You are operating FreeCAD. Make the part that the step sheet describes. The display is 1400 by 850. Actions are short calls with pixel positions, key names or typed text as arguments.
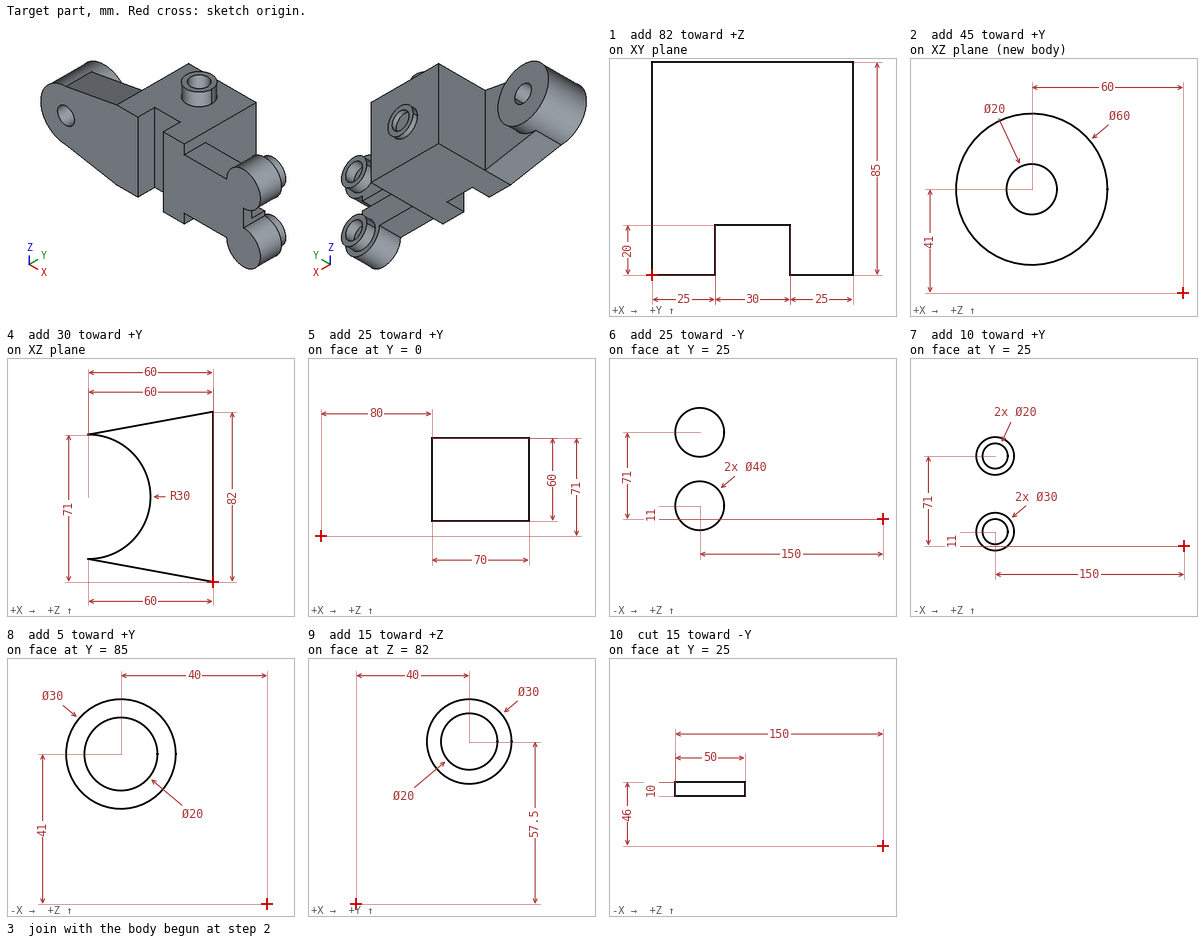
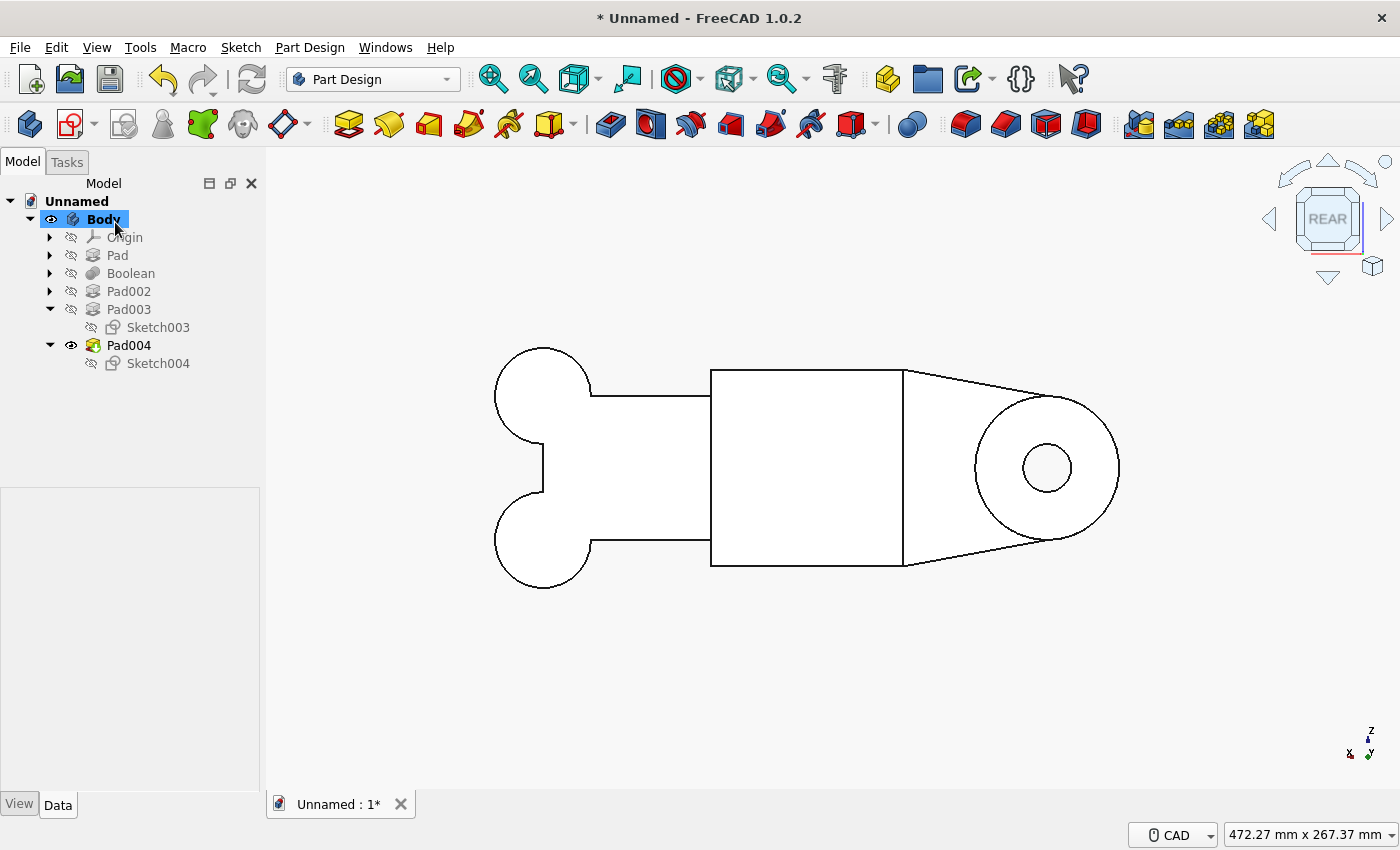
click(634, 467)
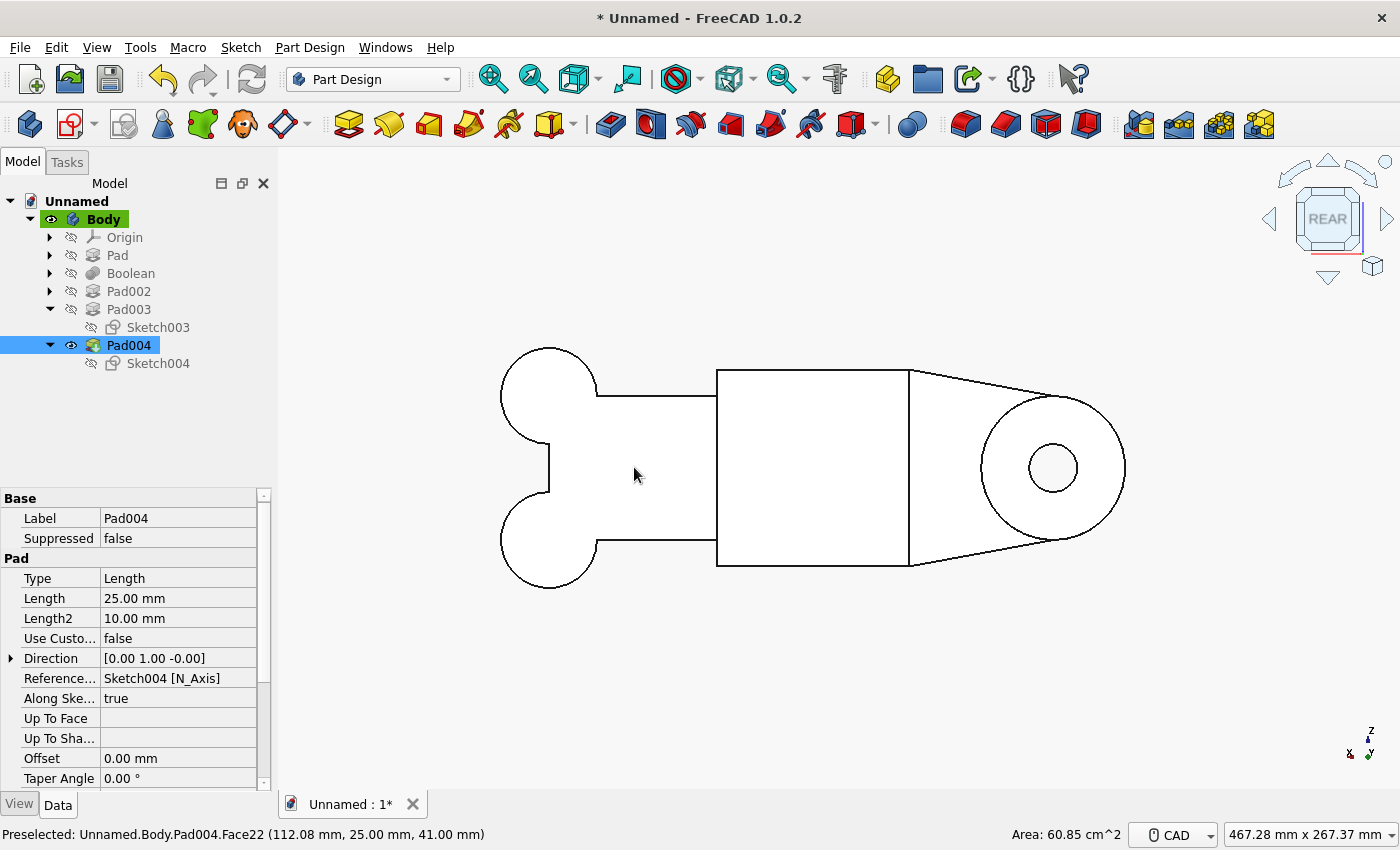
click(70, 124)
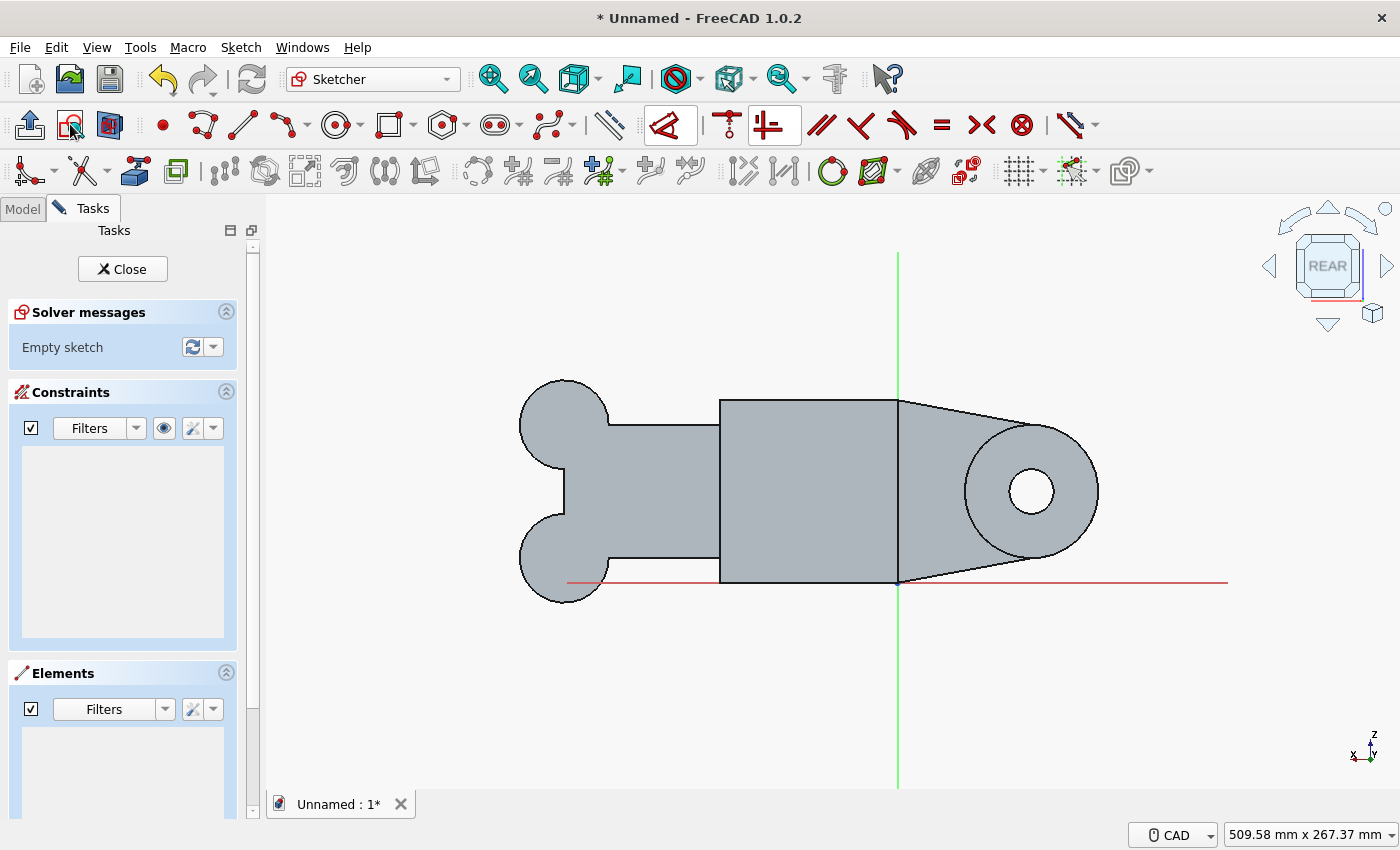
scroll(653, 492, up, 3)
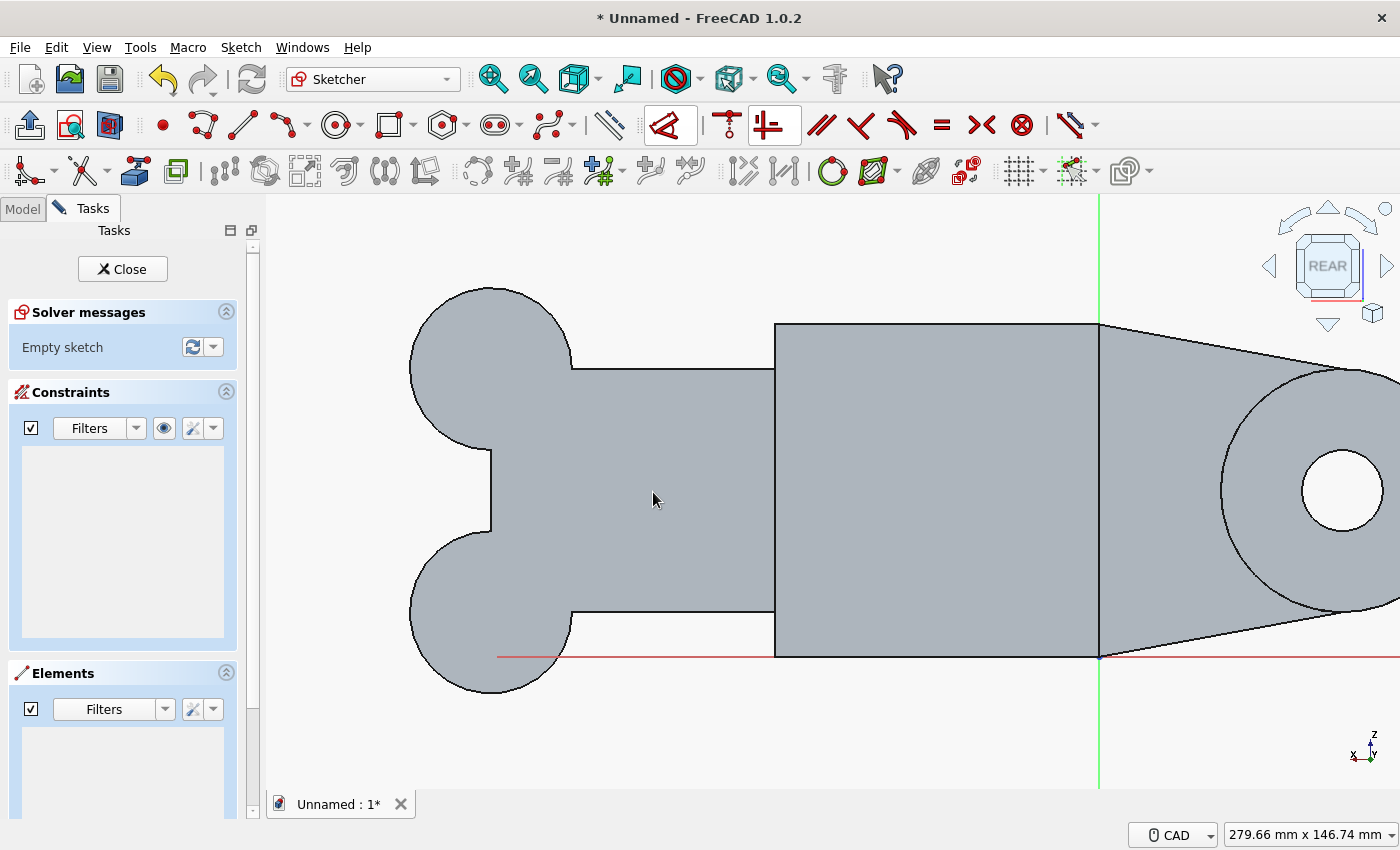
click(336, 126)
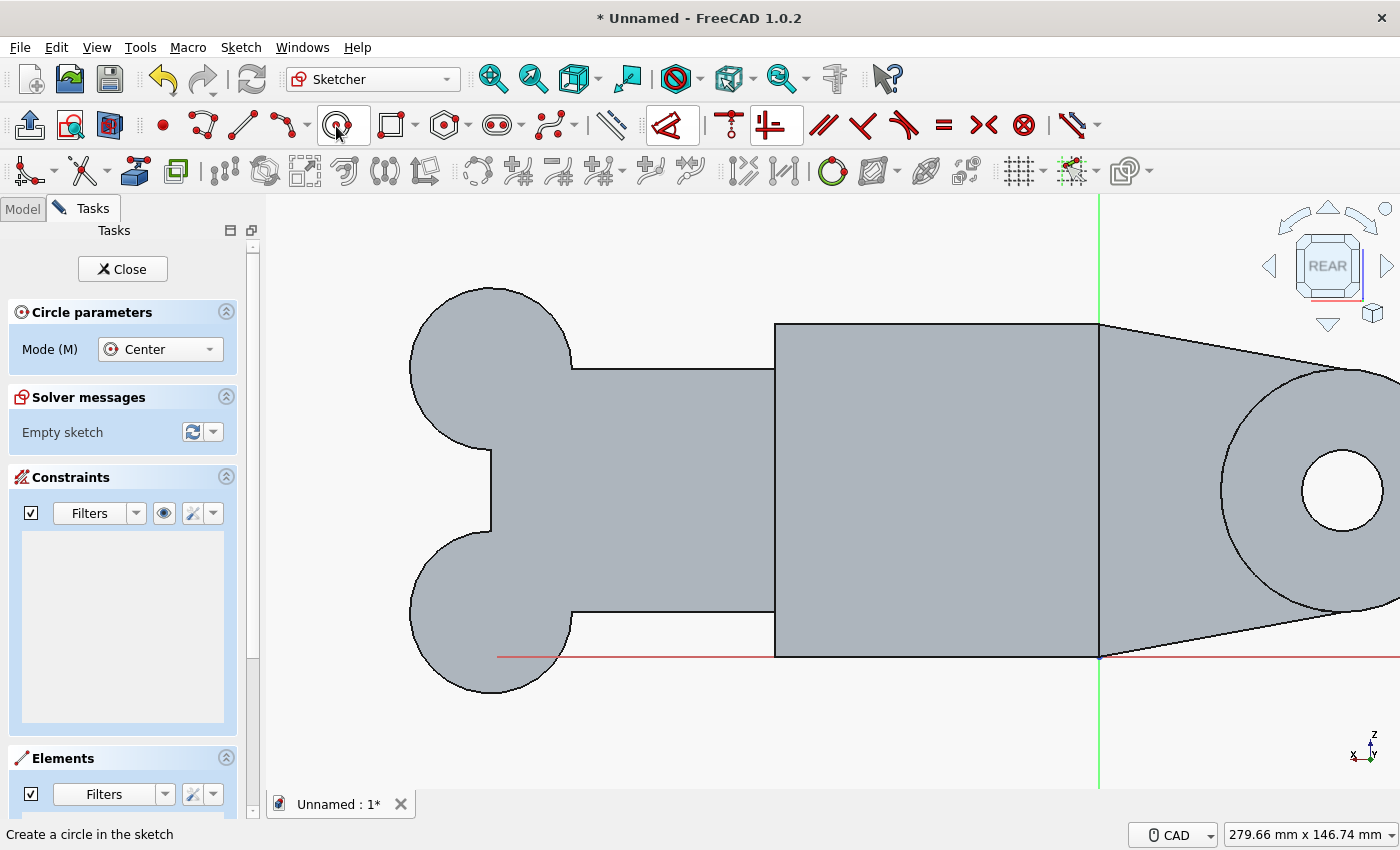
click(491, 612)
click(534, 569)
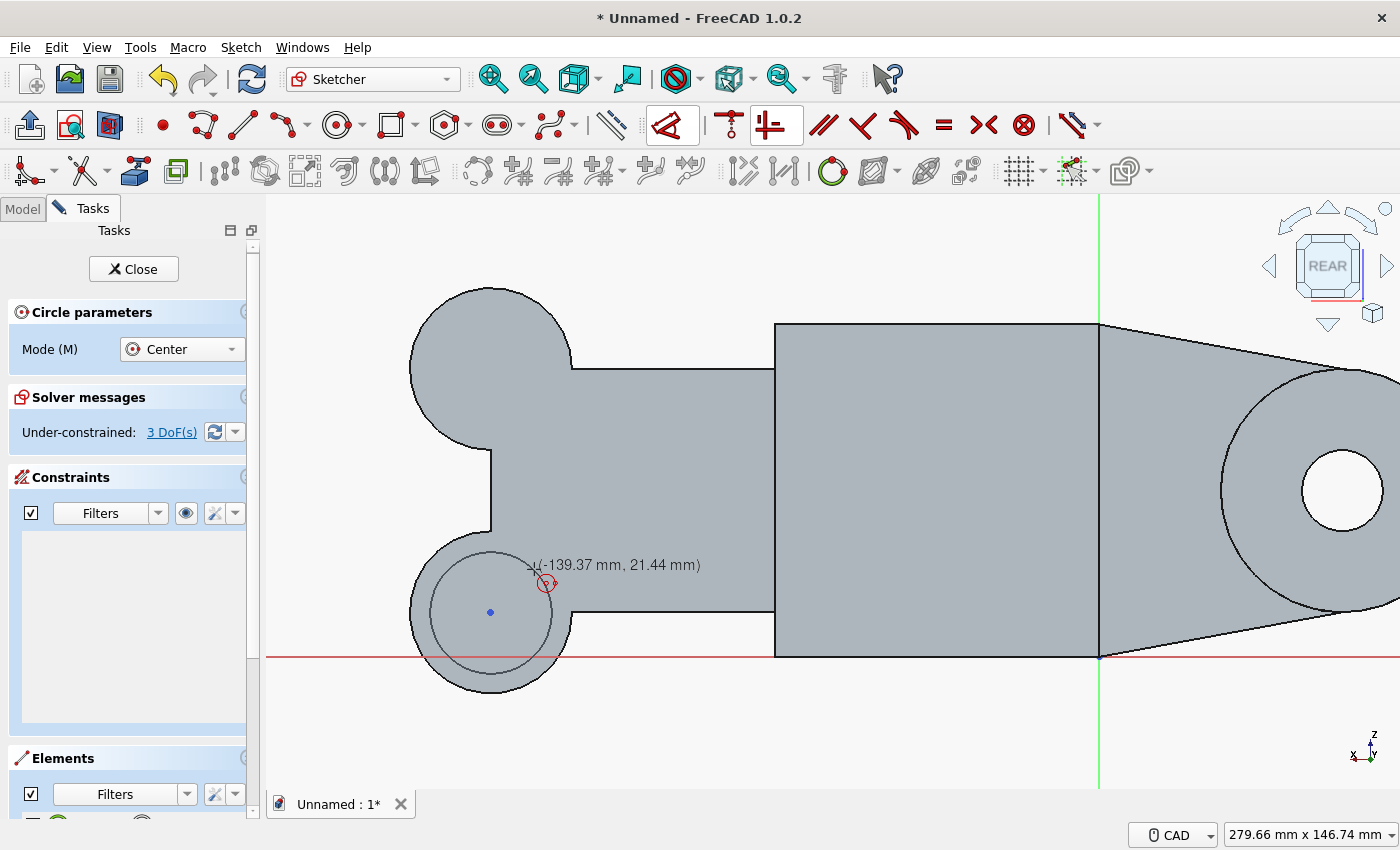
click(491, 369)
click(534, 326)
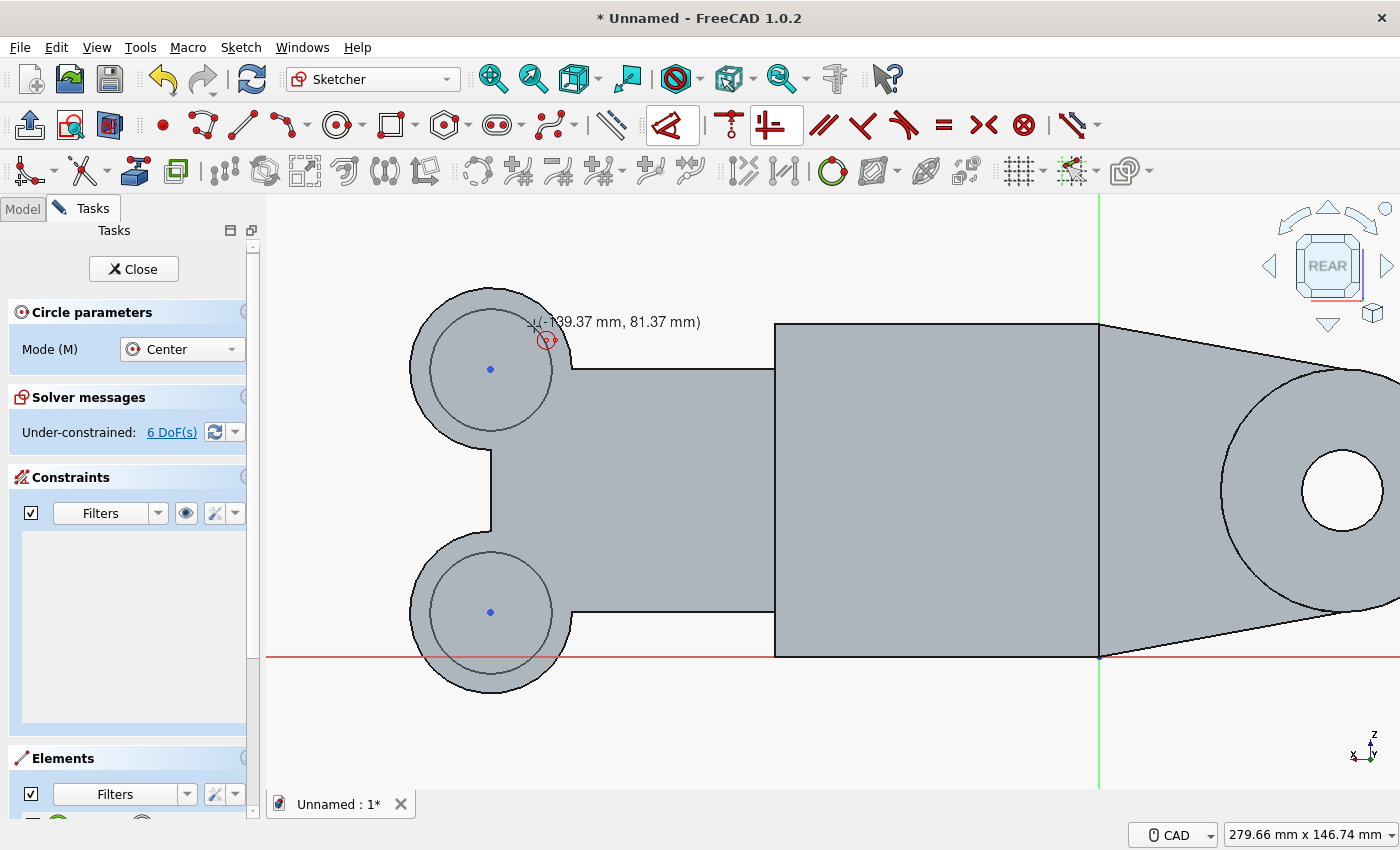
click(491, 613)
click(520, 584)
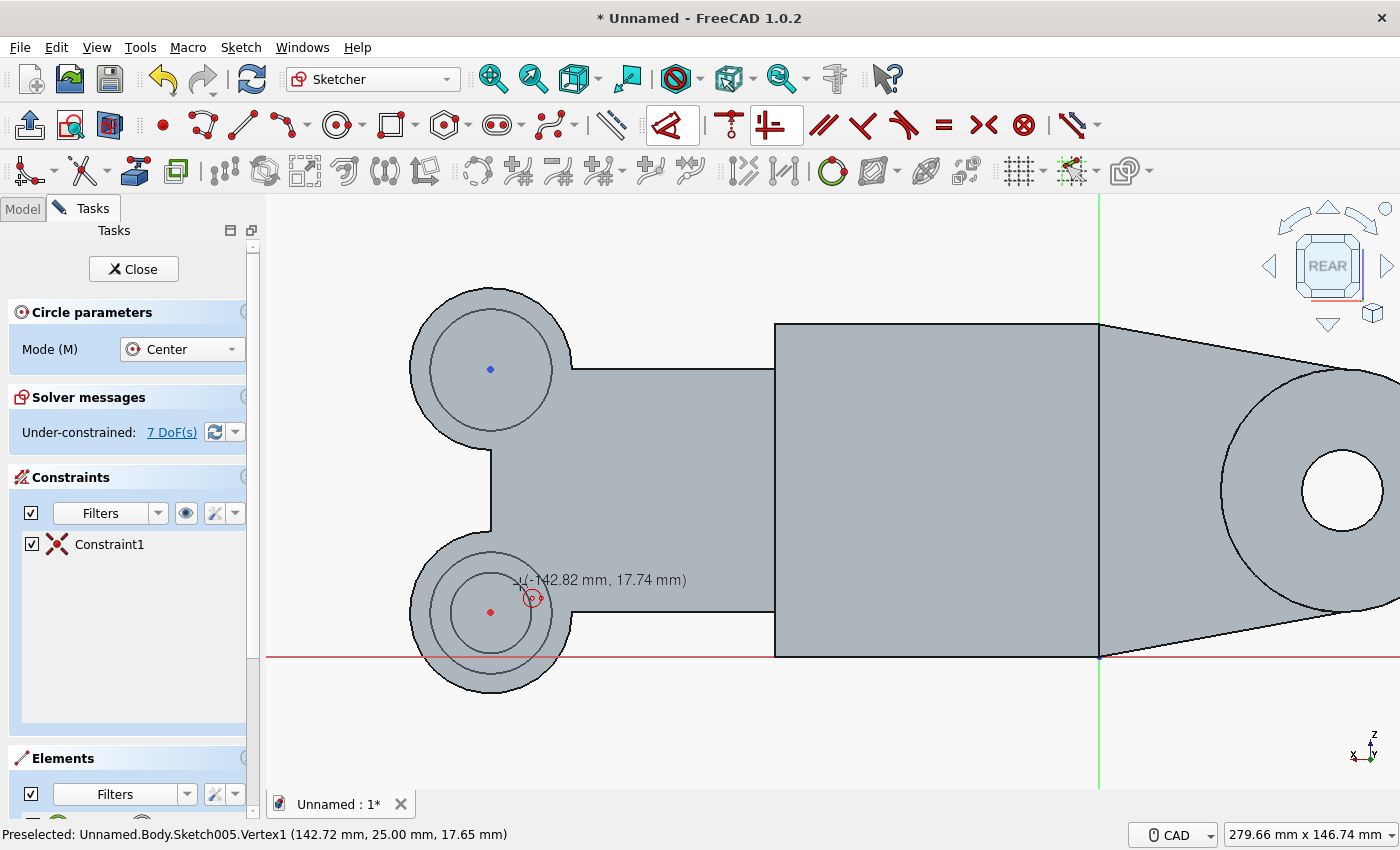
click(491, 370)
click(520, 340)
key(Escape)